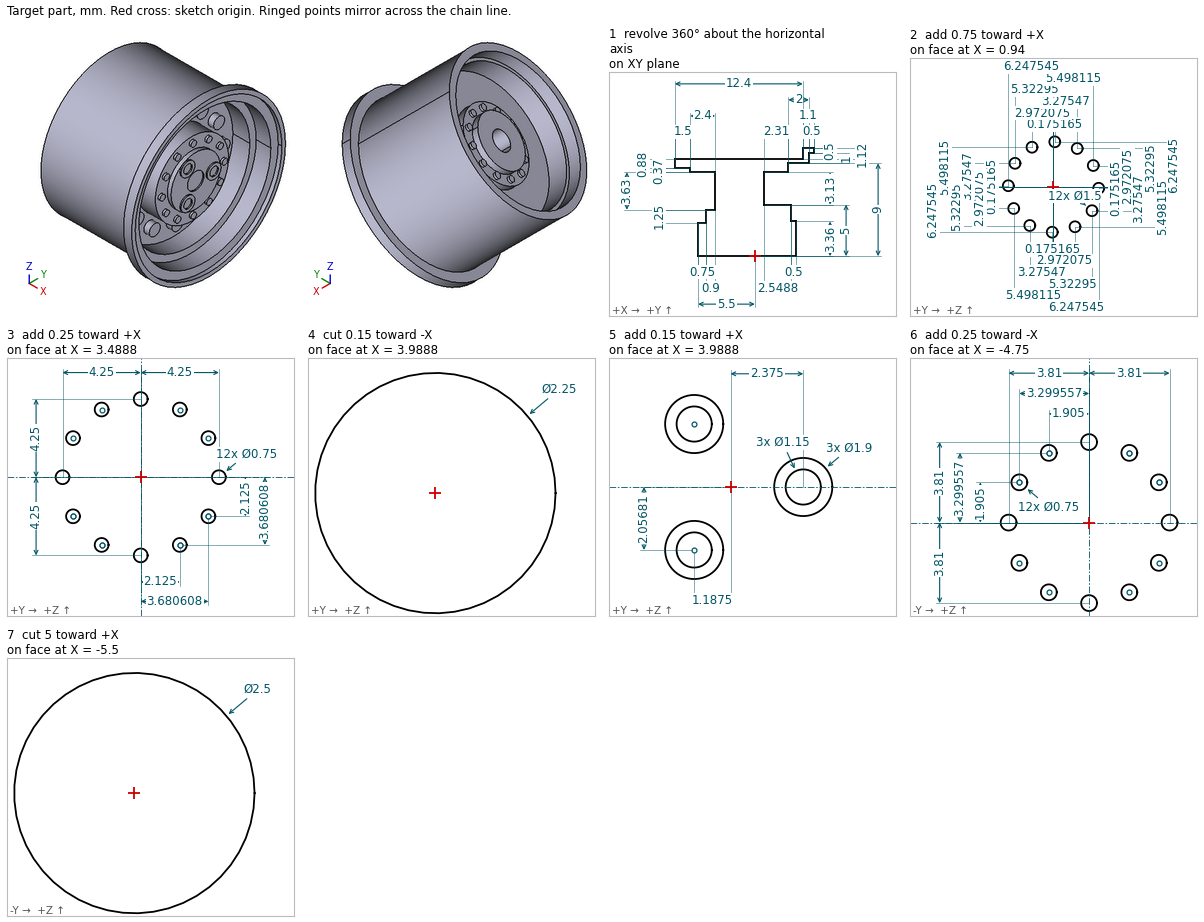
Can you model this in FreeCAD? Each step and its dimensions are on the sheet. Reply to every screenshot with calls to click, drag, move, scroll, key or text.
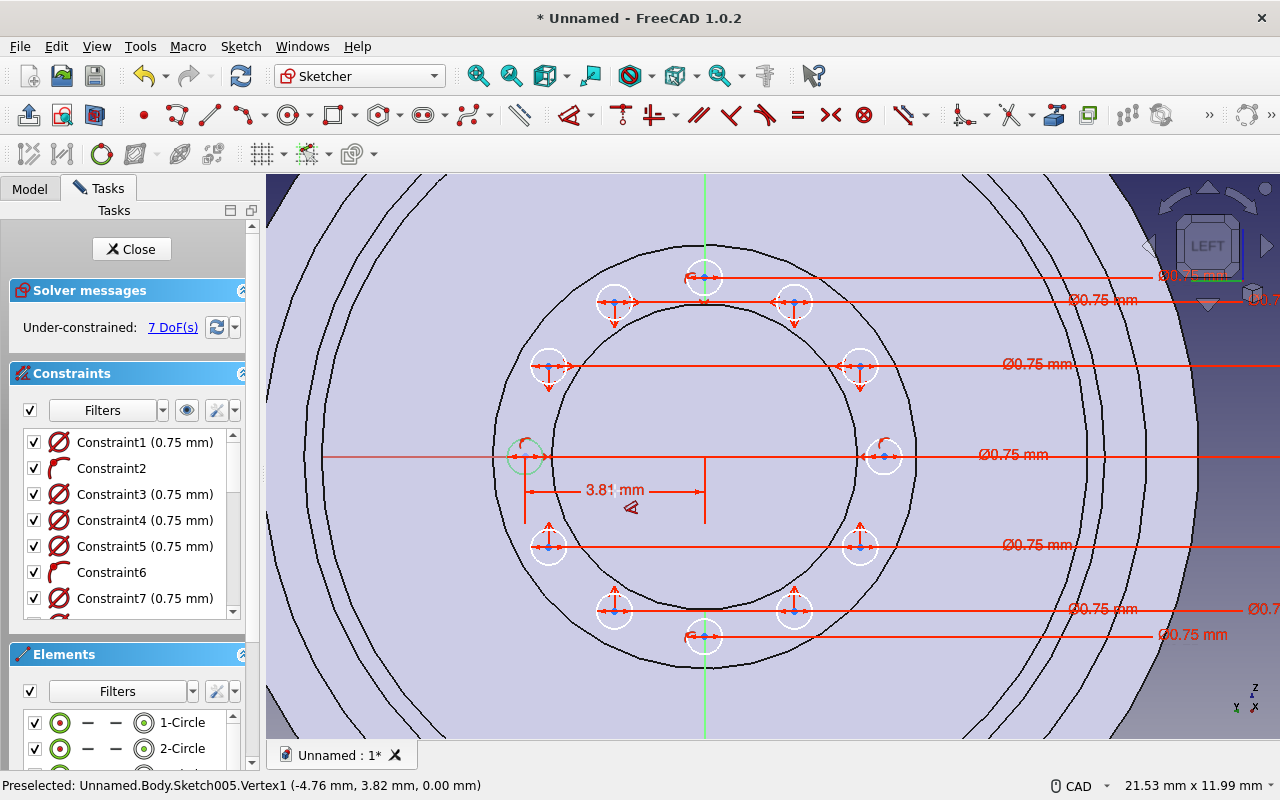
click(705, 278)
click(739, 367)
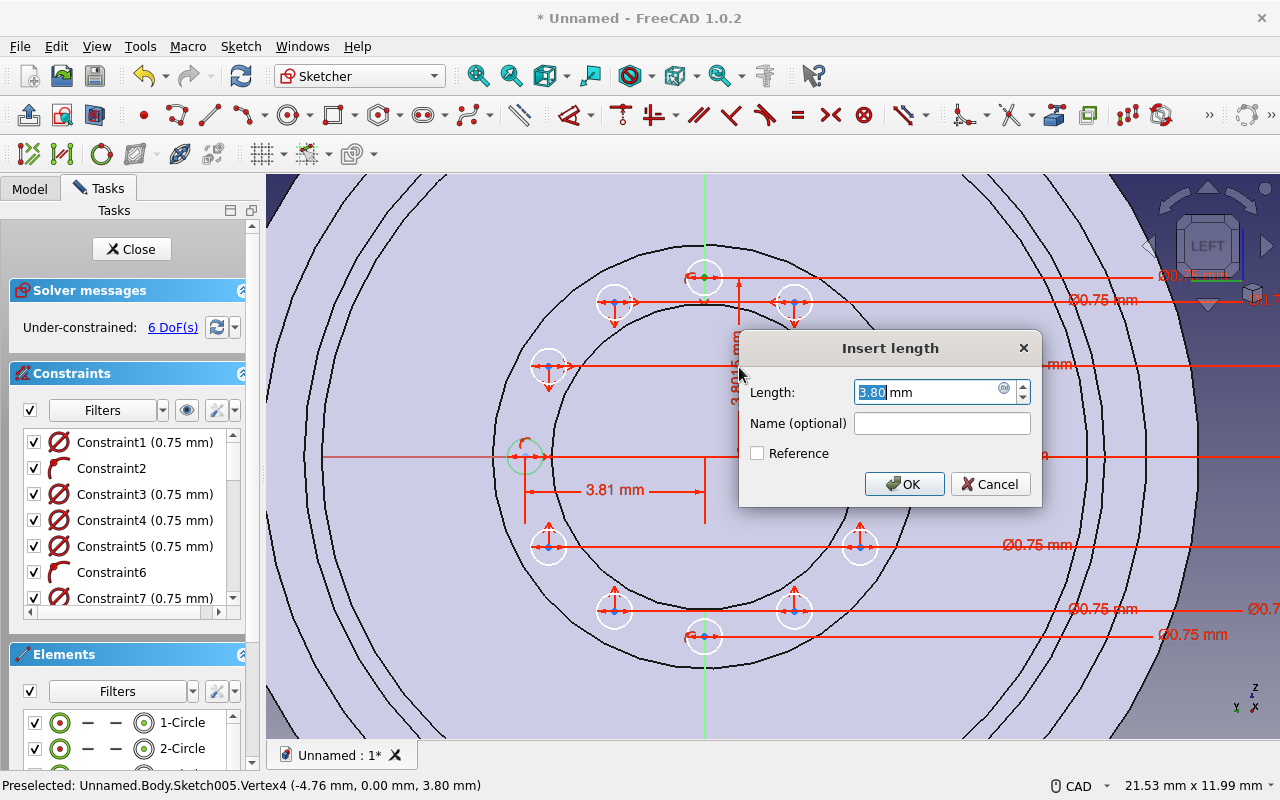
text(3.81)
key(Return)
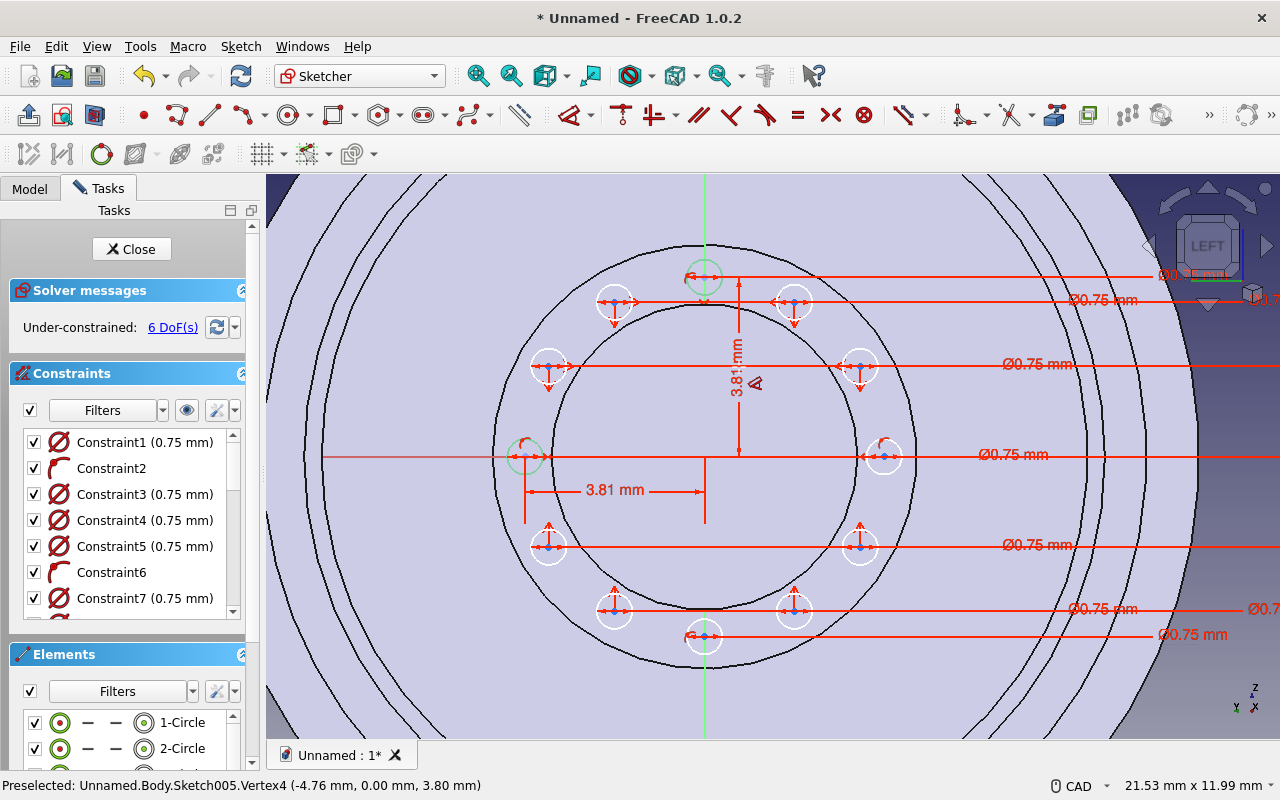
click(884, 457)
click(794, 491)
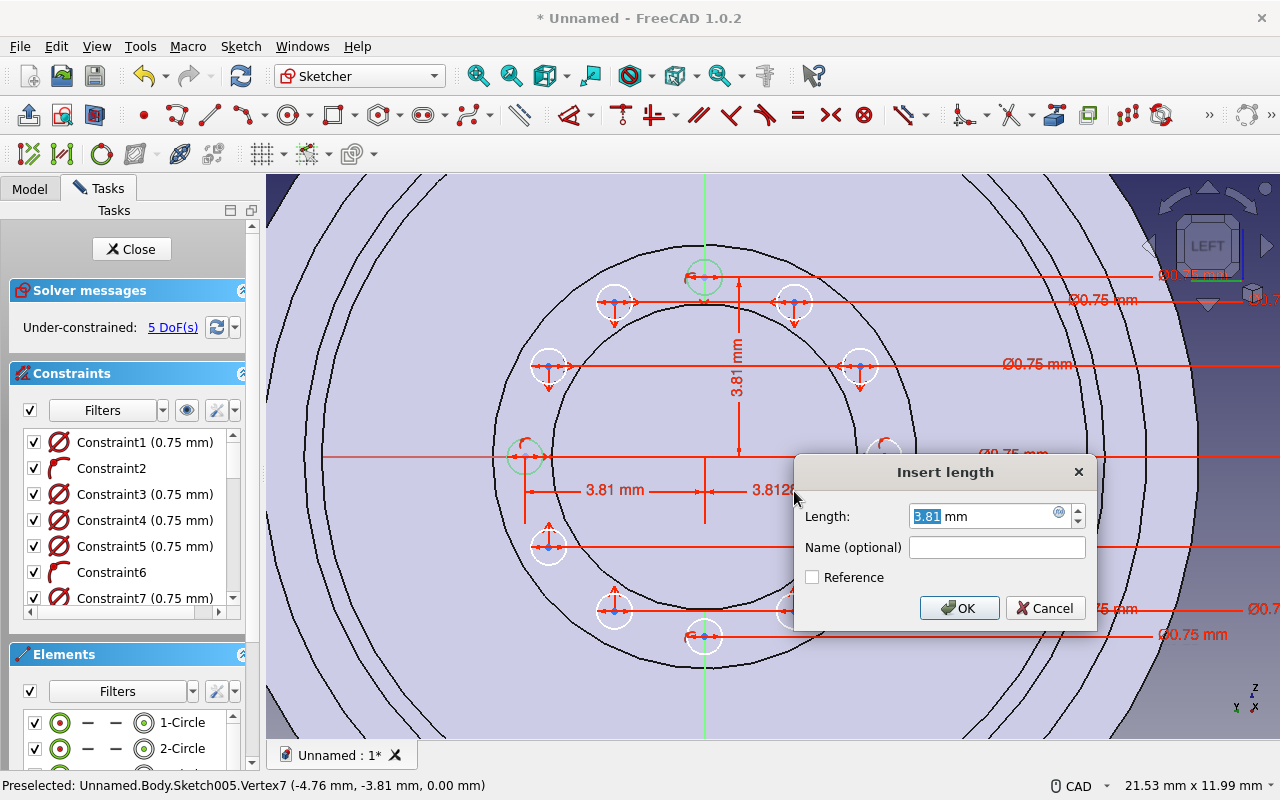
text(3.81)
key(Return)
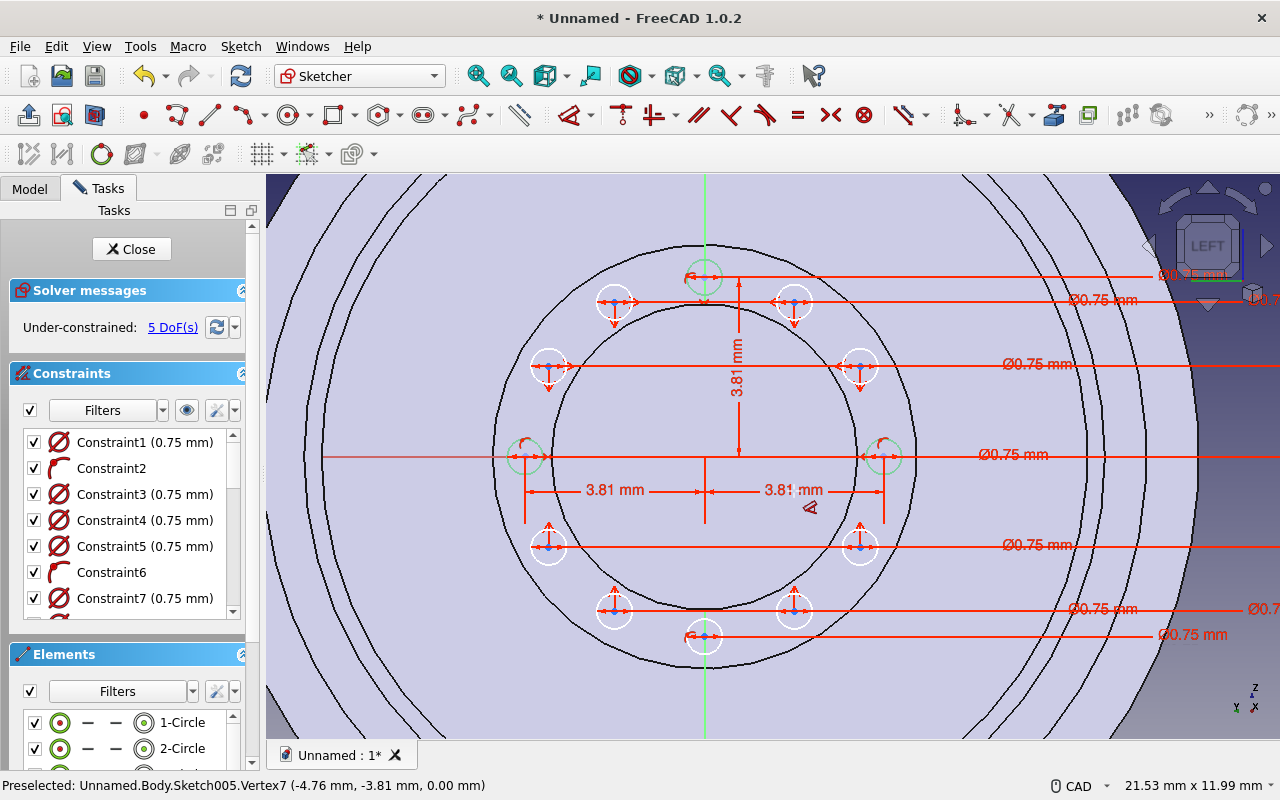
click(705, 637)
click(739, 547)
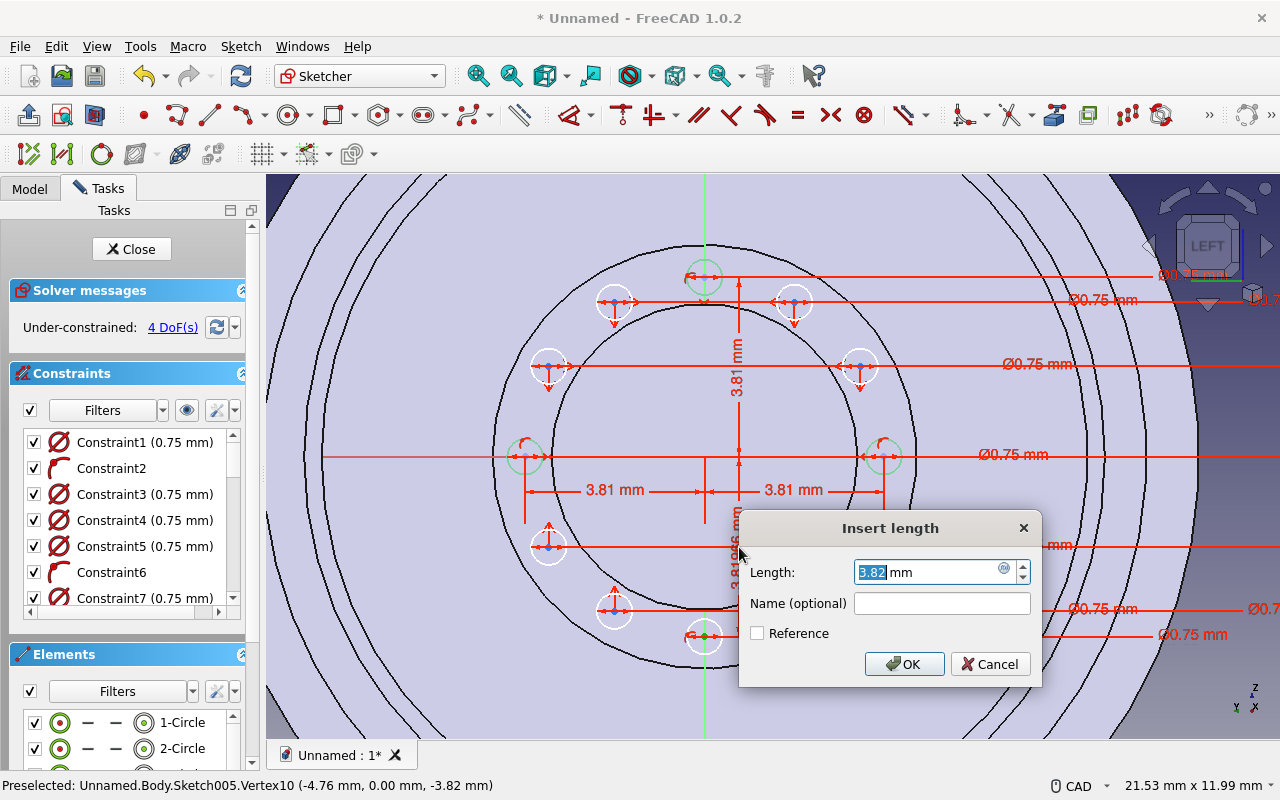
text(3.81)
key(Return)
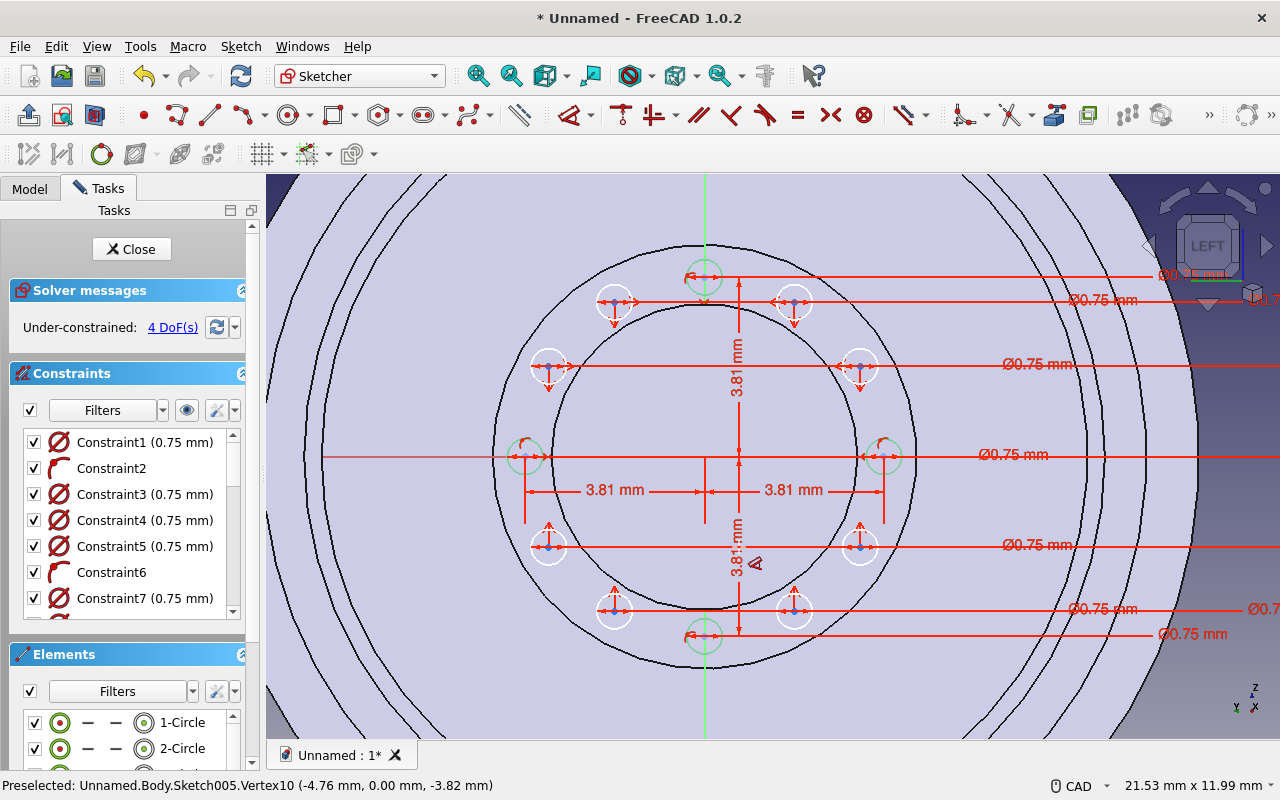
click(549, 366)
click(515, 412)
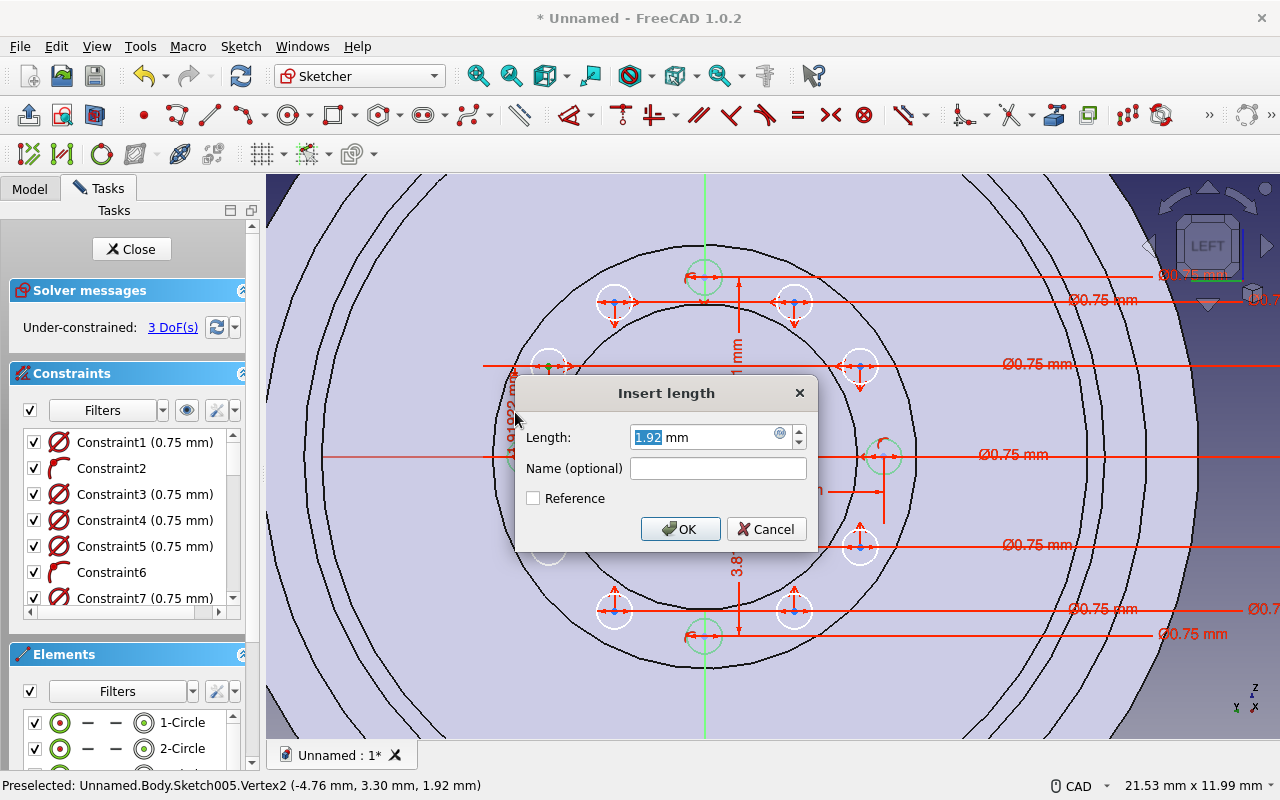
text(1.905)
key(Return)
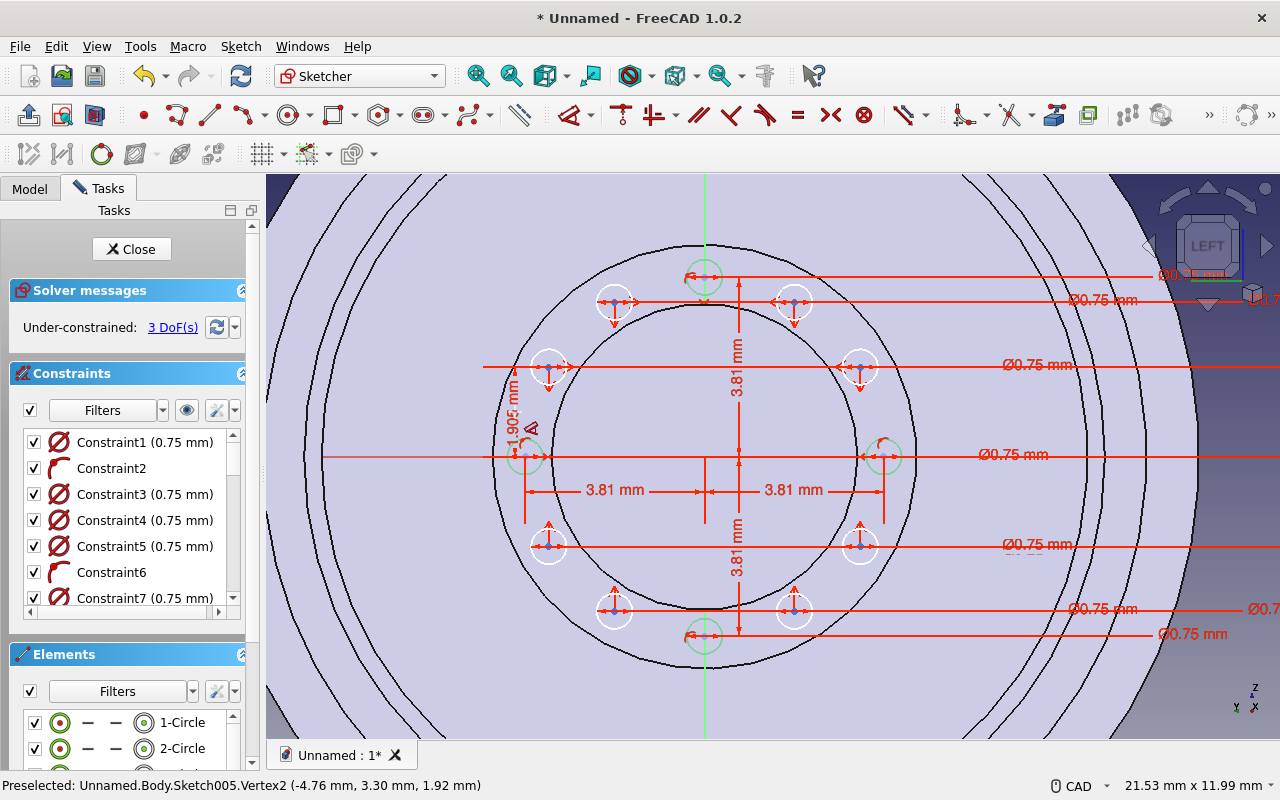
click(615, 302)
click(660, 268)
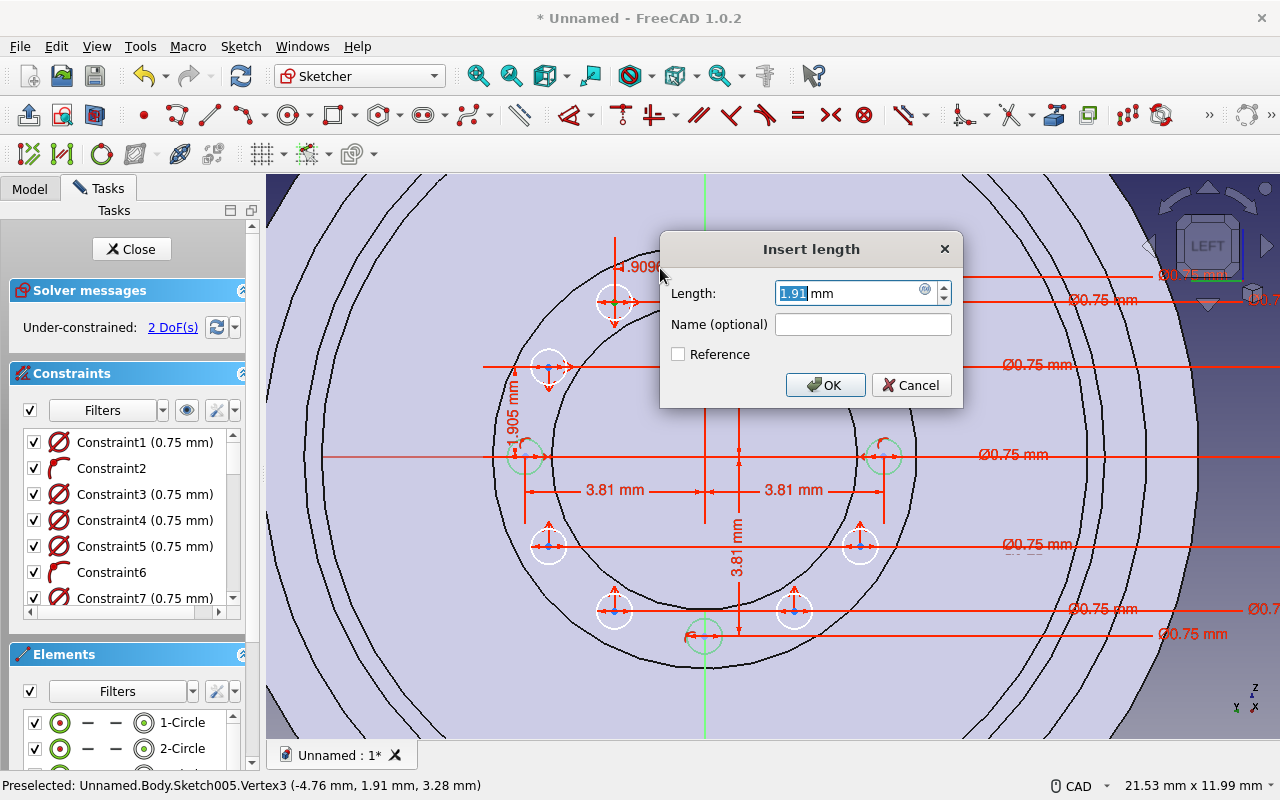
text(1.905)
key(Return)